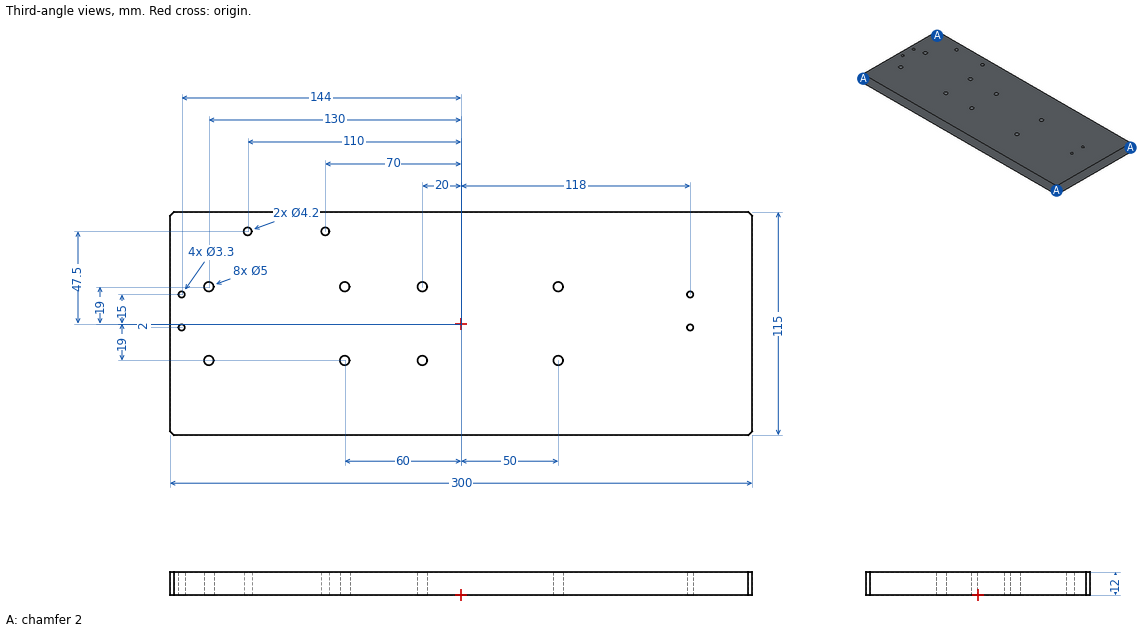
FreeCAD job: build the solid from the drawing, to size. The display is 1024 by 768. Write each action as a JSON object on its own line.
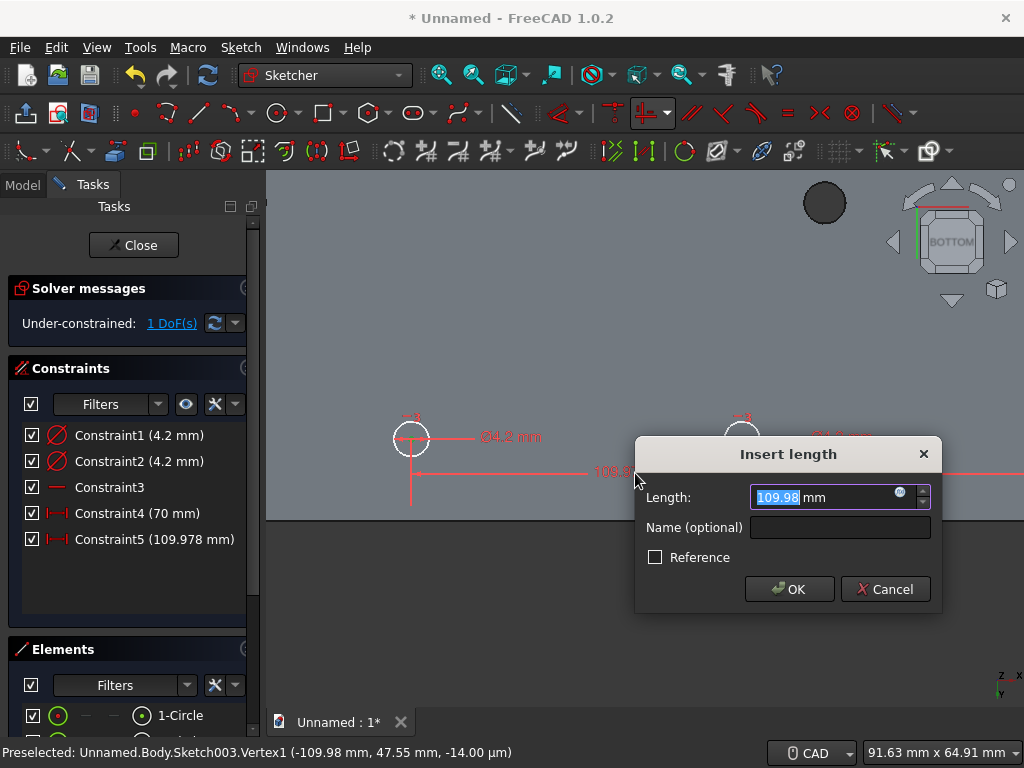
{"action": "type", "text": "110"}
{"action": "key", "text": "Return"}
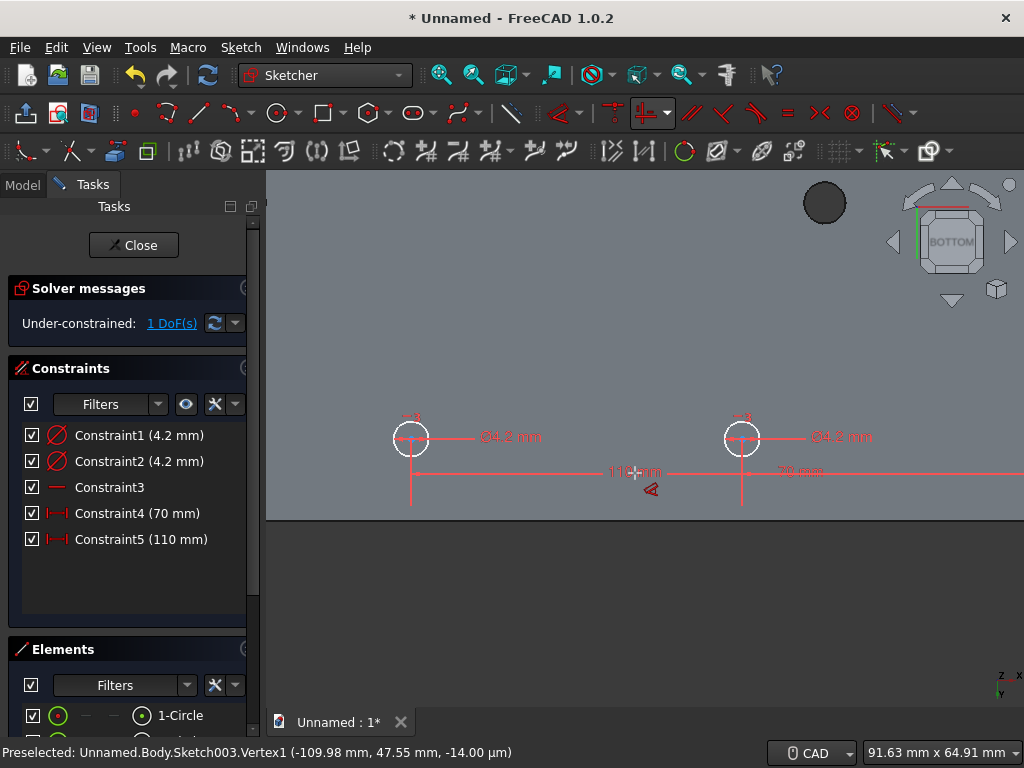
{"action": "left_click", "coordinate": [411, 439]}
{"action": "left_click", "coordinate": [377, 319]}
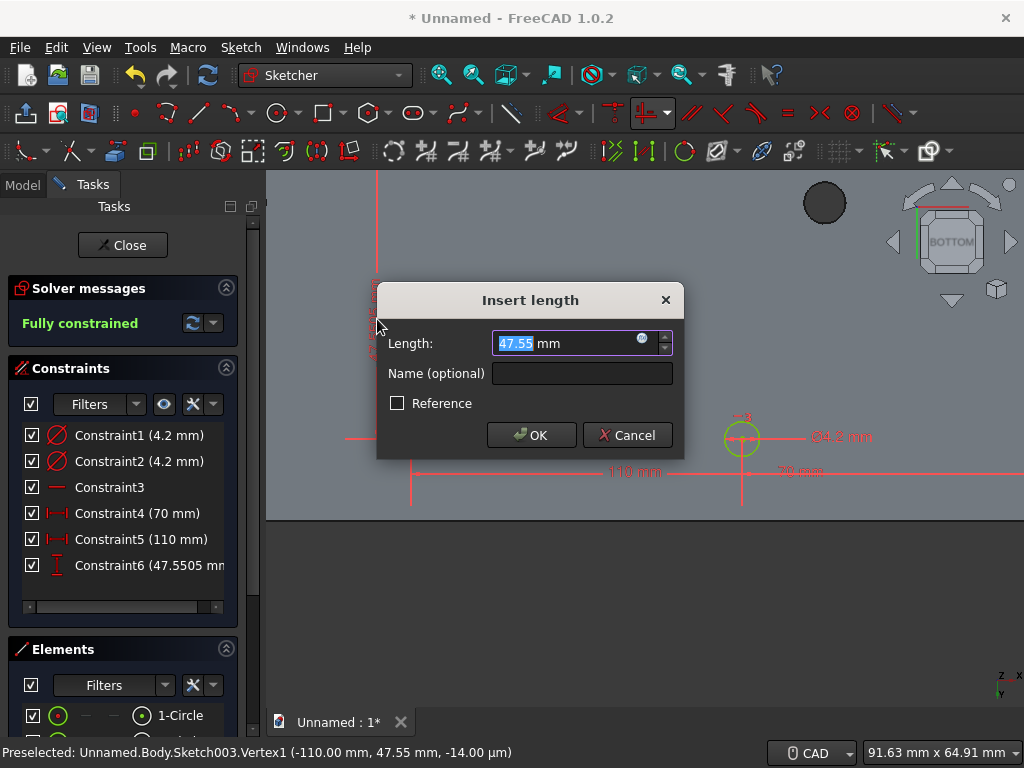
{"action": "type", "text": "47.5"}
{"action": "key", "text": "Return"}
{"action": "key", "text": "Escape"}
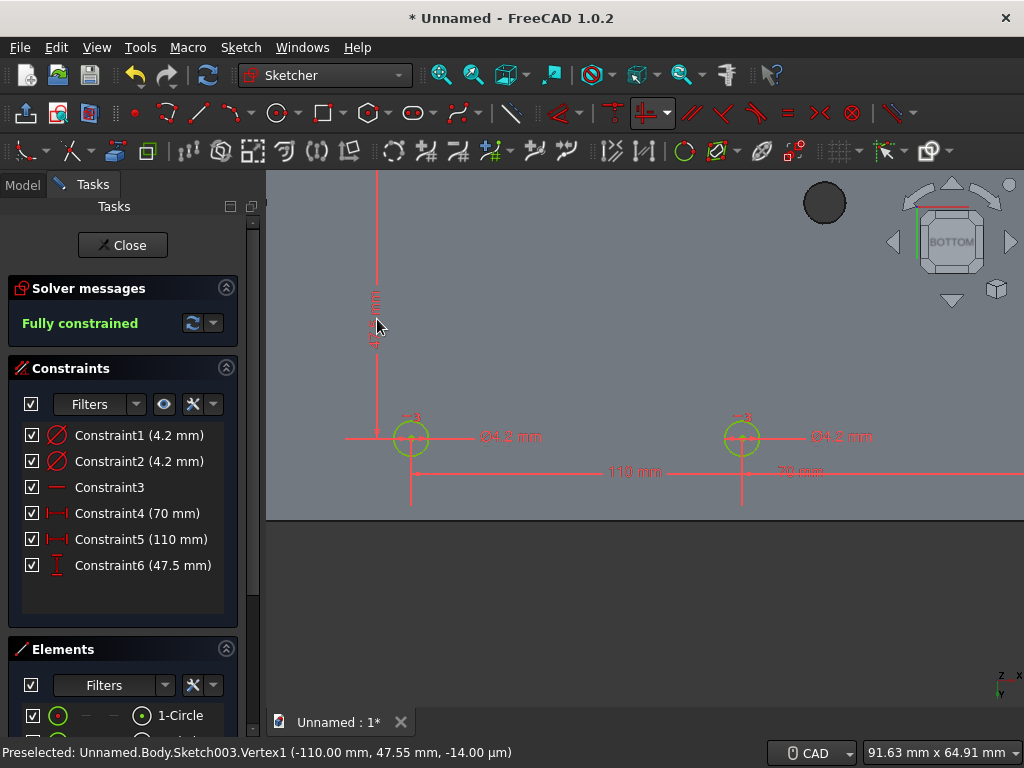
{"action": "left_click", "coordinate": [123, 245]}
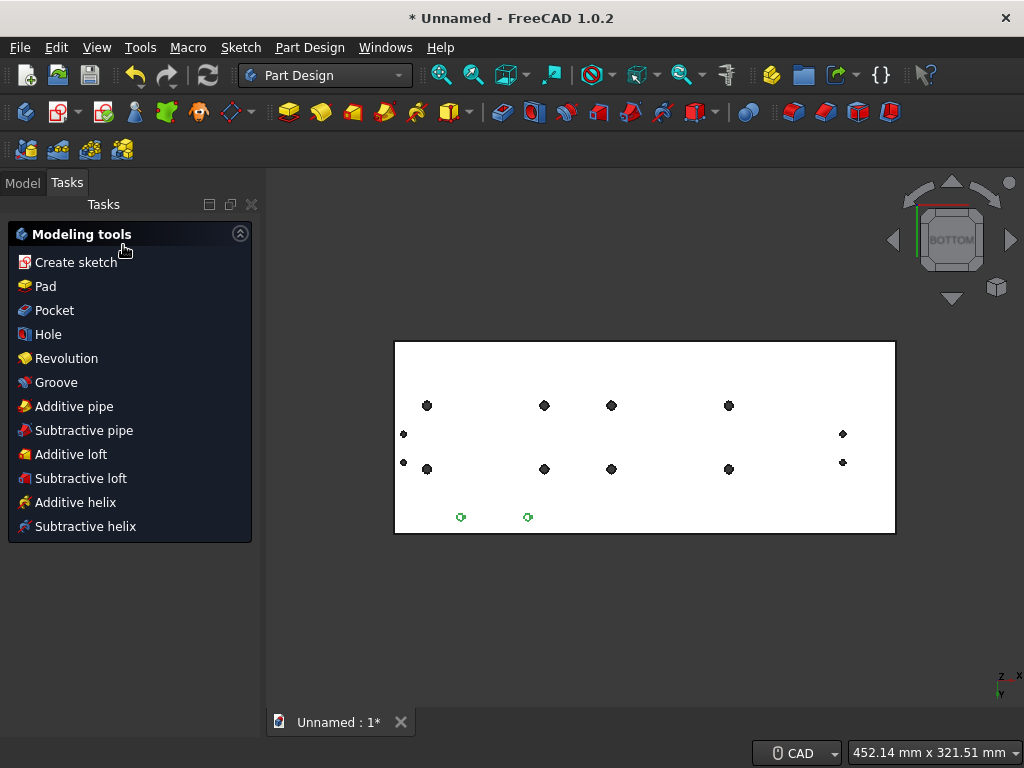
{"action": "left_click", "coordinate": [504, 112]}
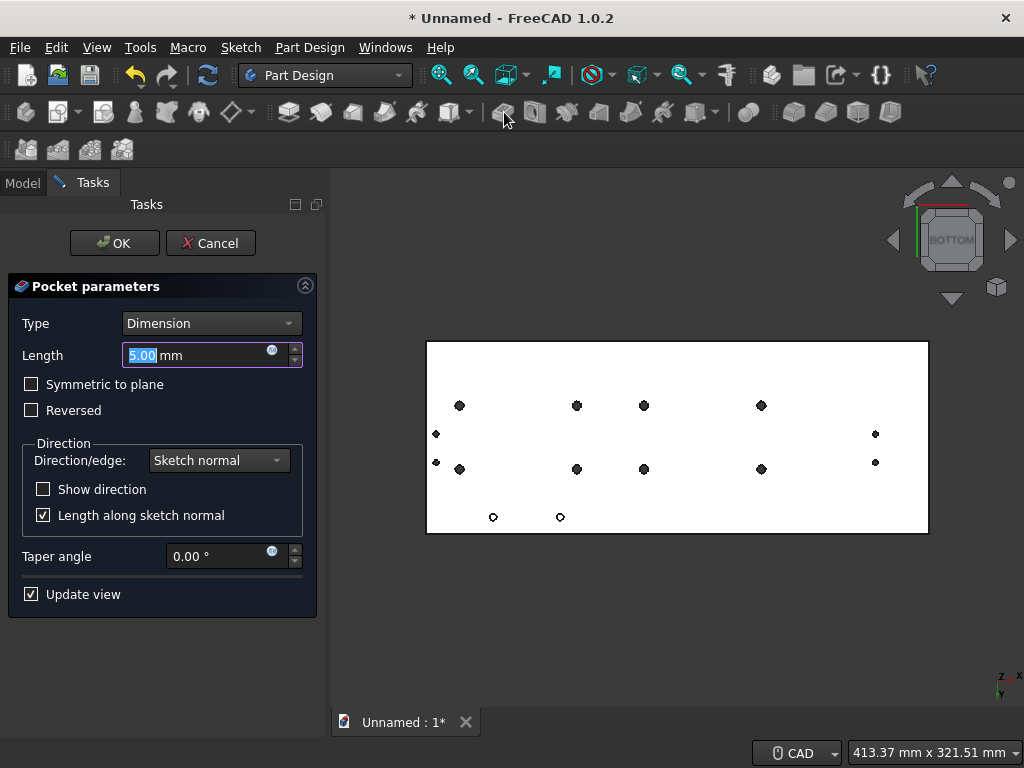
{"action": "left_click", "coordinate": [212, 324]}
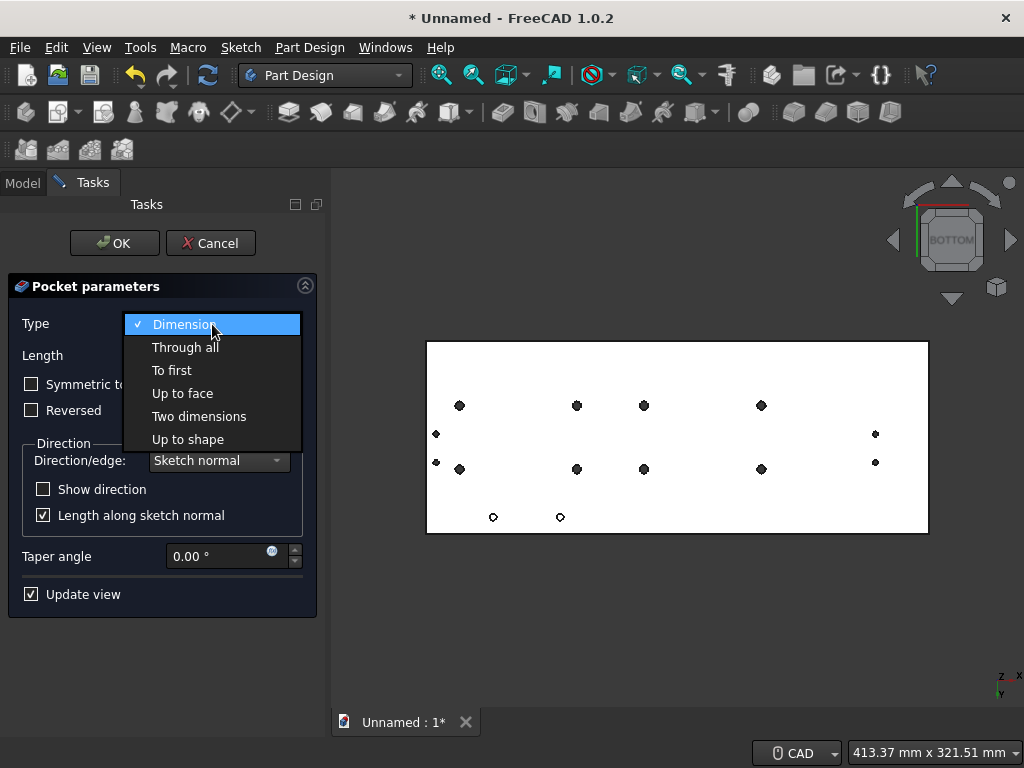
{"action": "left_click", "coordinate": [212, 348]}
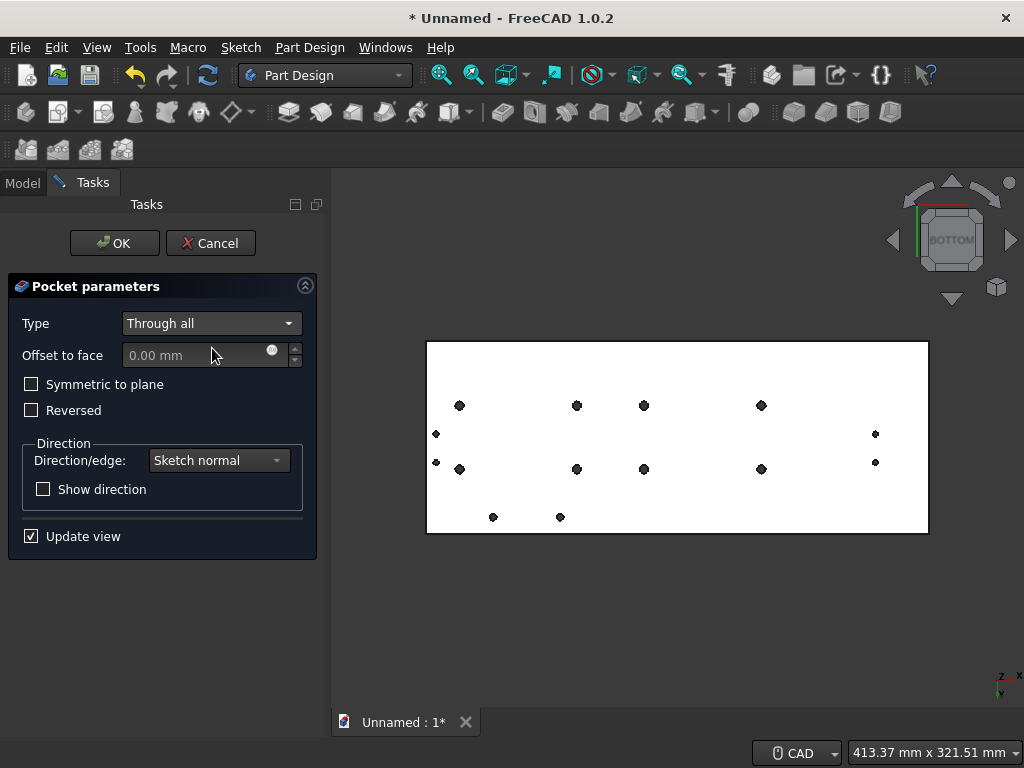
{"action": "left_click", "coordinate": [115, 243]}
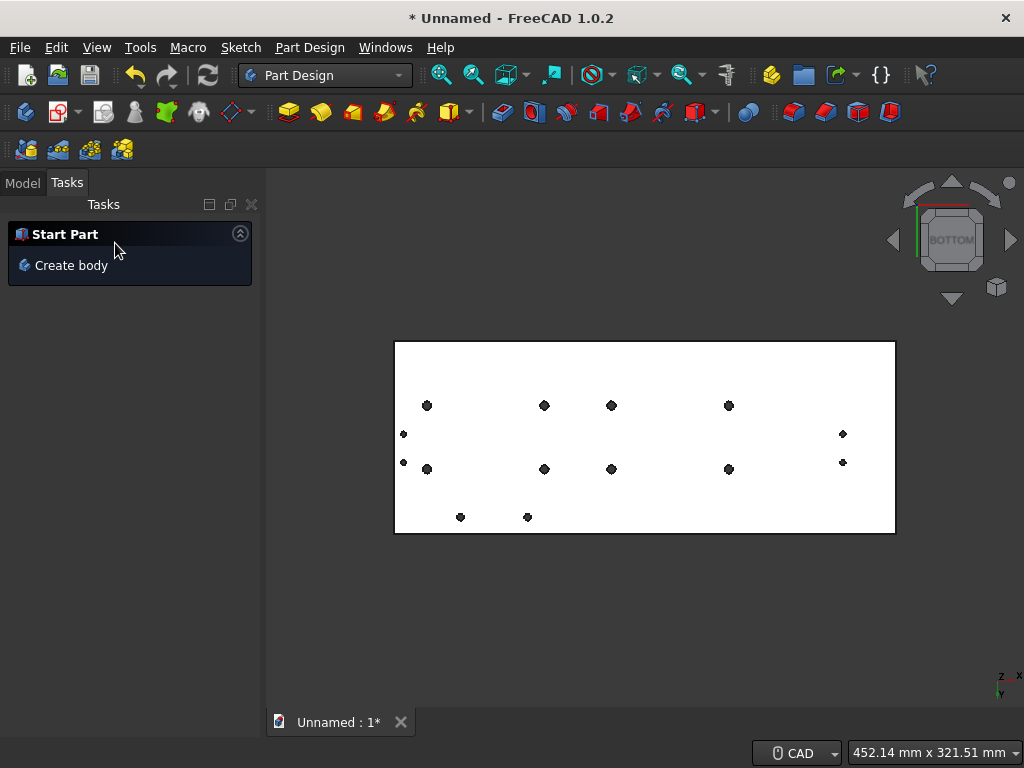
{"action": "key", "text": "0"}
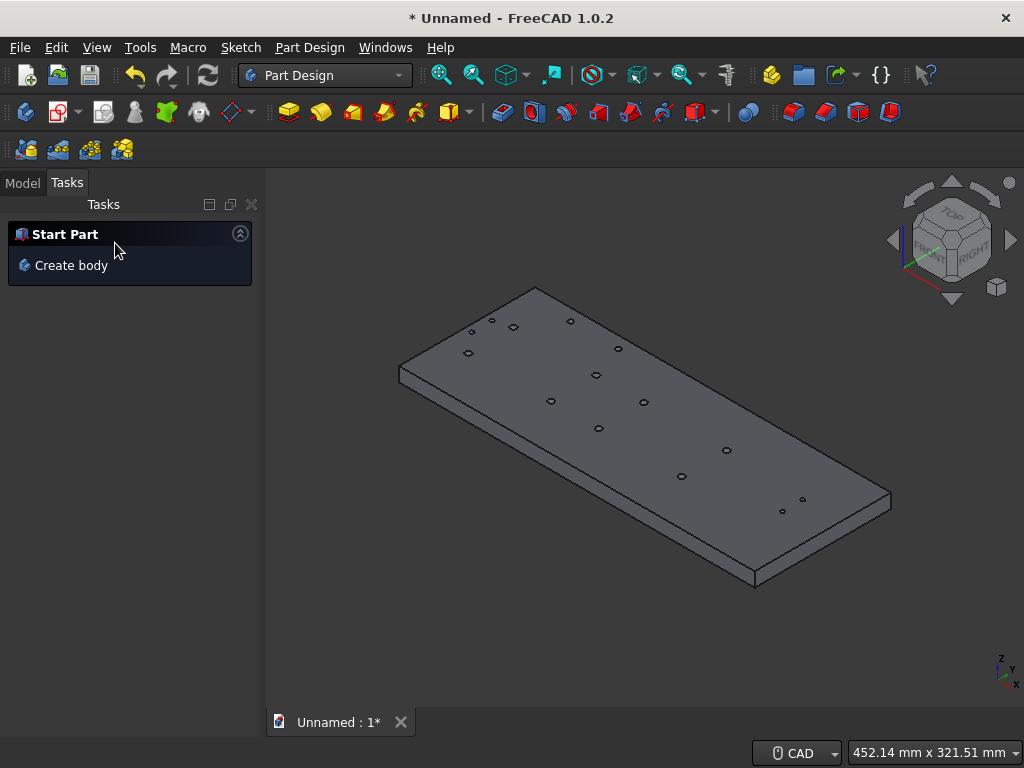
{"action": "left_click", "coordinate": [755, 579]}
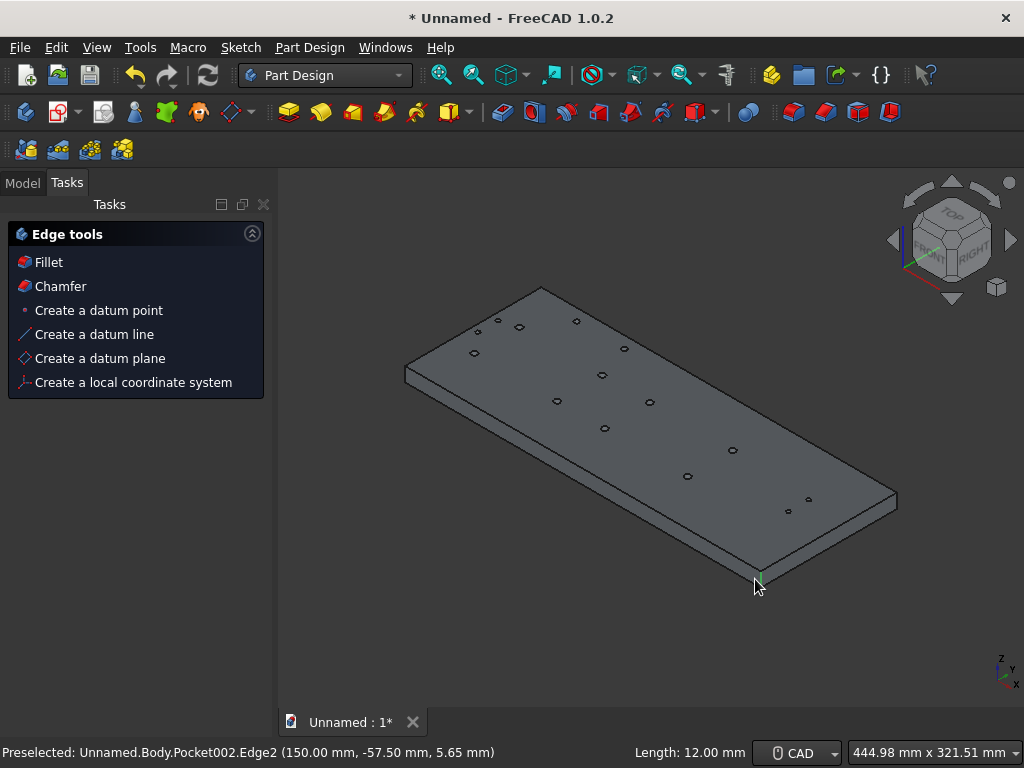
{"action": "scroll", "coordinate": [405, 373], "scroll_direction": "up", "scroll_amount": 4}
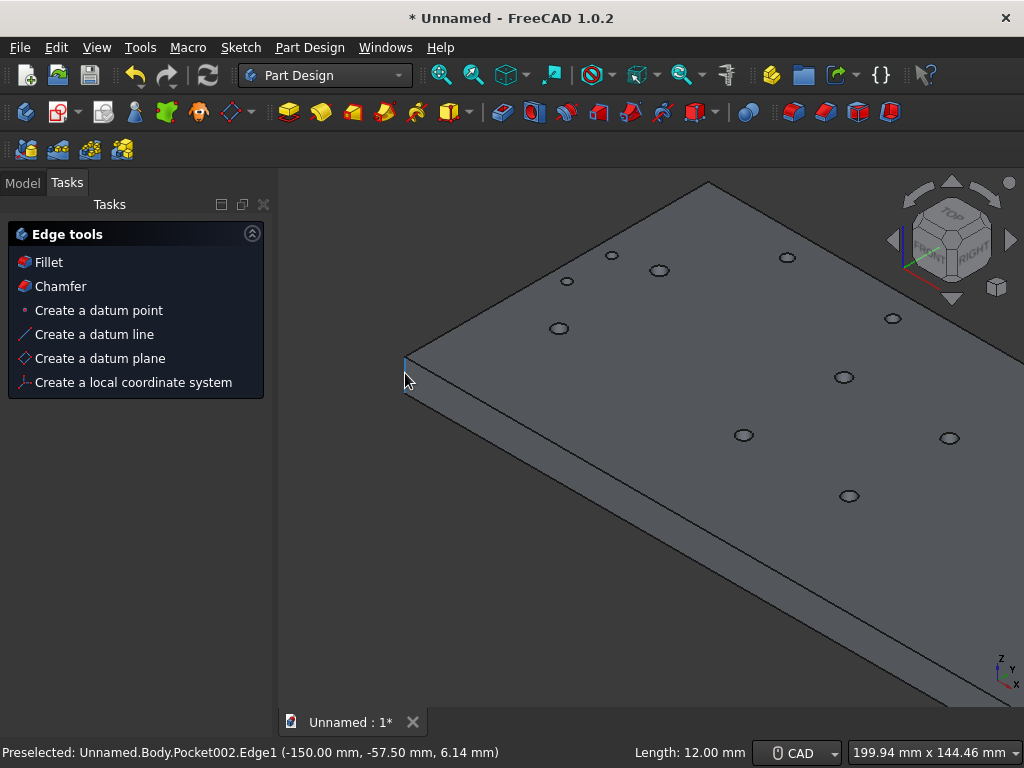
{"action": "key", "text": "v f"}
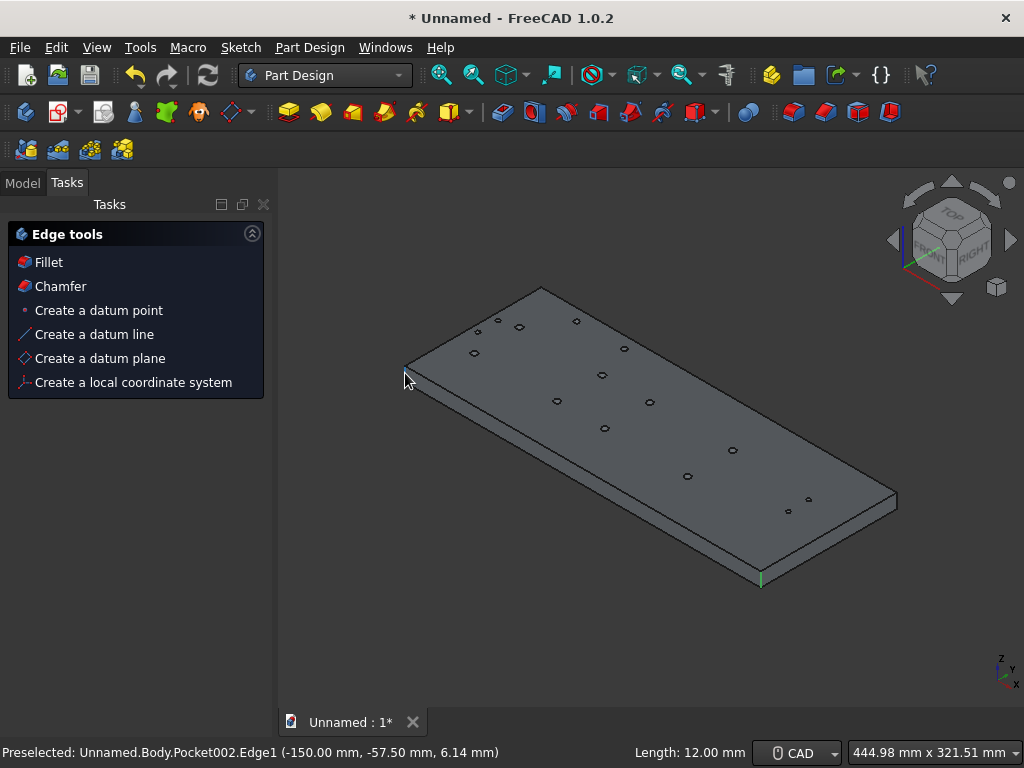
{"action": "key", "text": "2"}